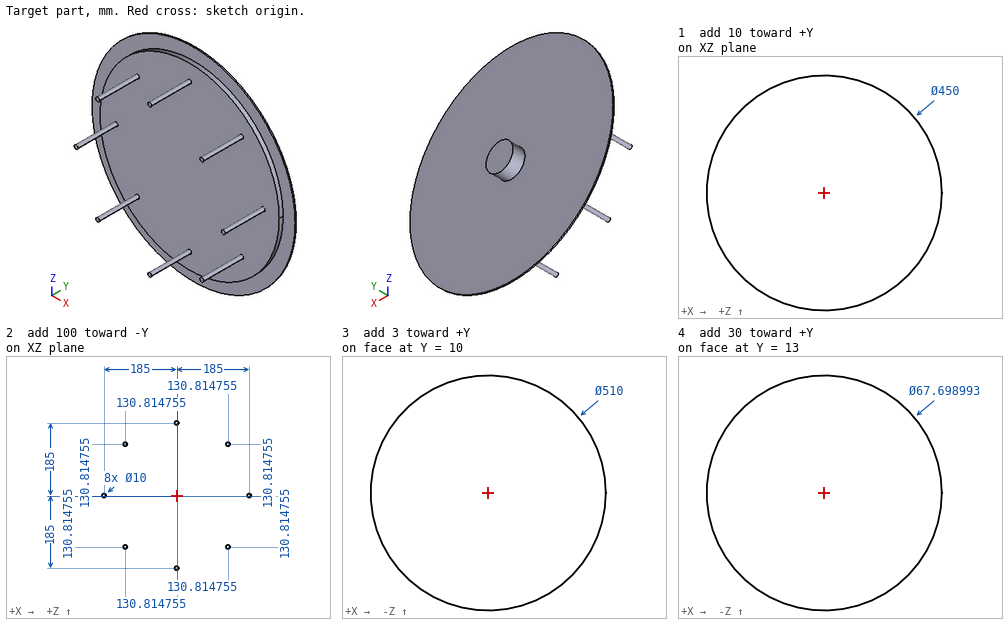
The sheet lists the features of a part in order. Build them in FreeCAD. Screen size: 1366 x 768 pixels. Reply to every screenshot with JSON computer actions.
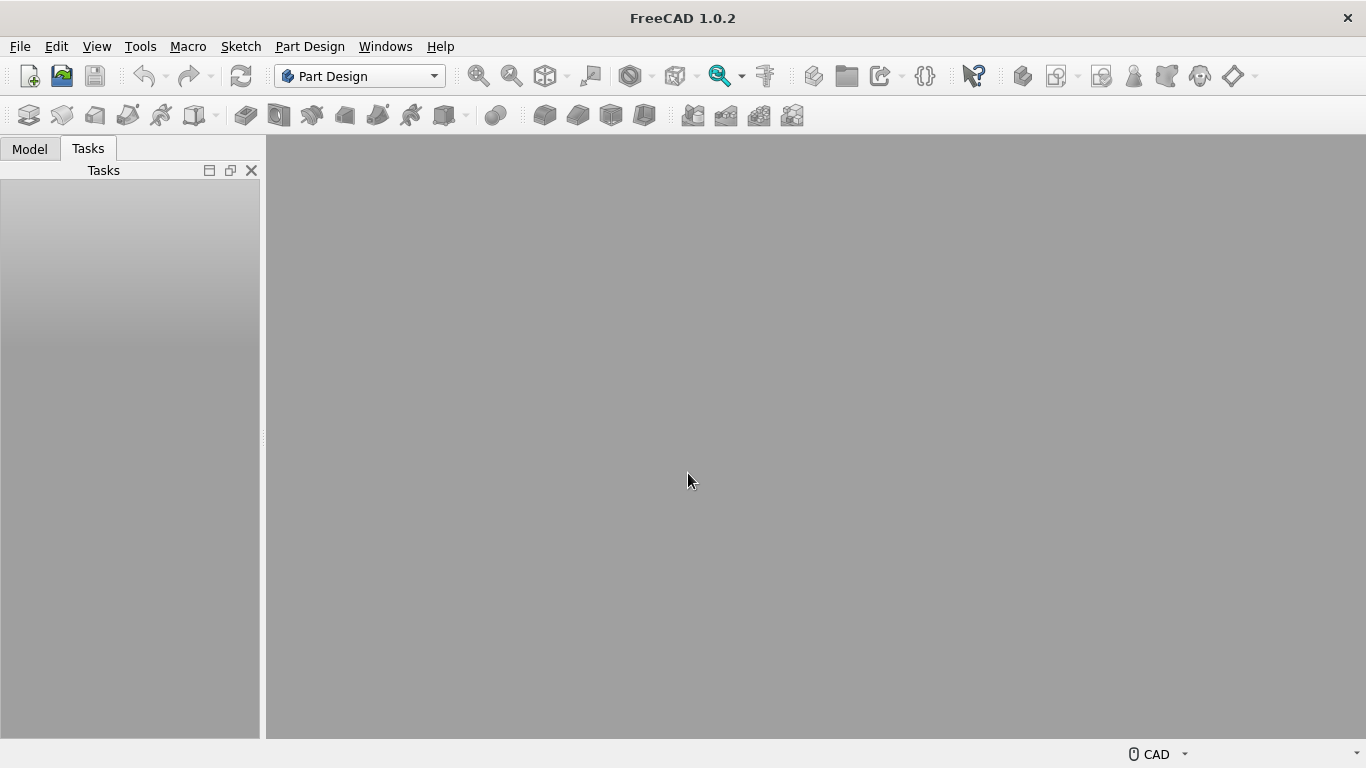
{"action": "left_click", "coordinate": [29, 76]}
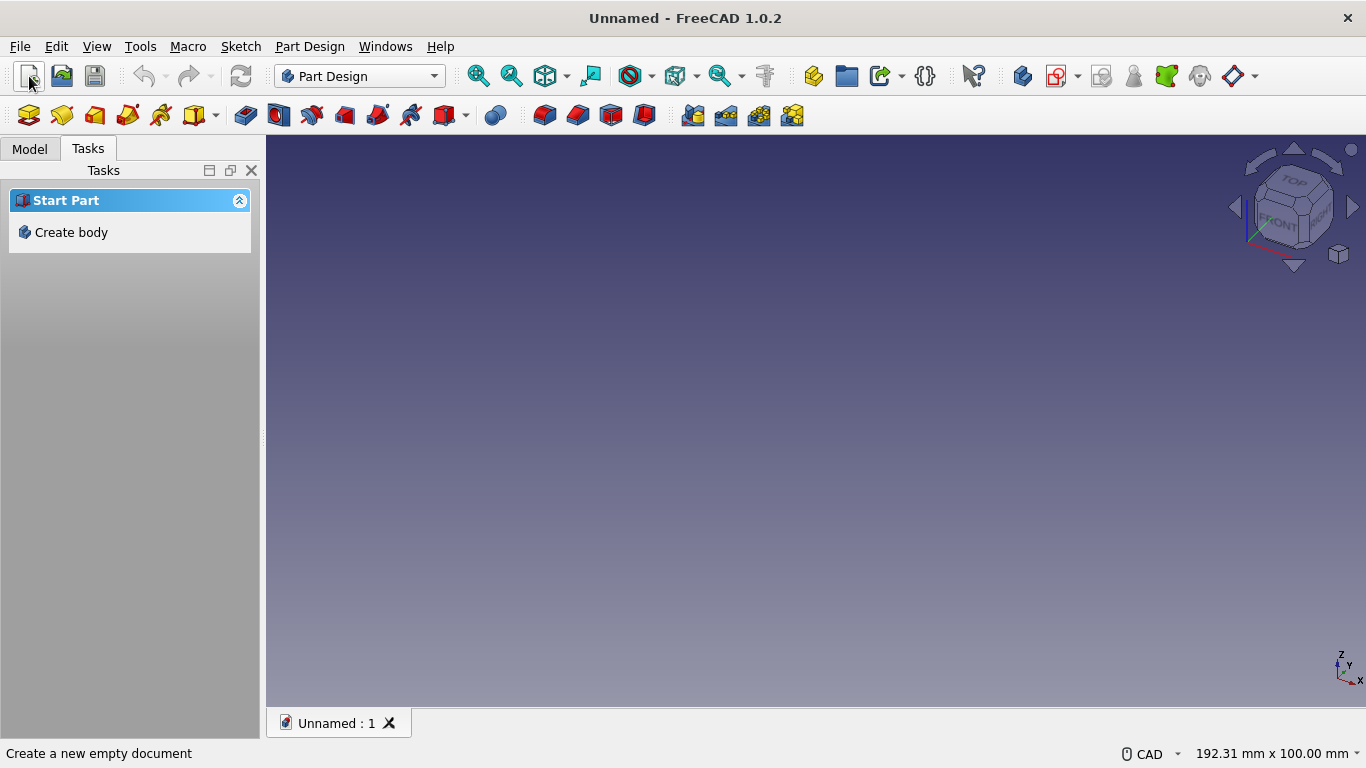
{"action": "left_click", "coordinate": [1056, 76]}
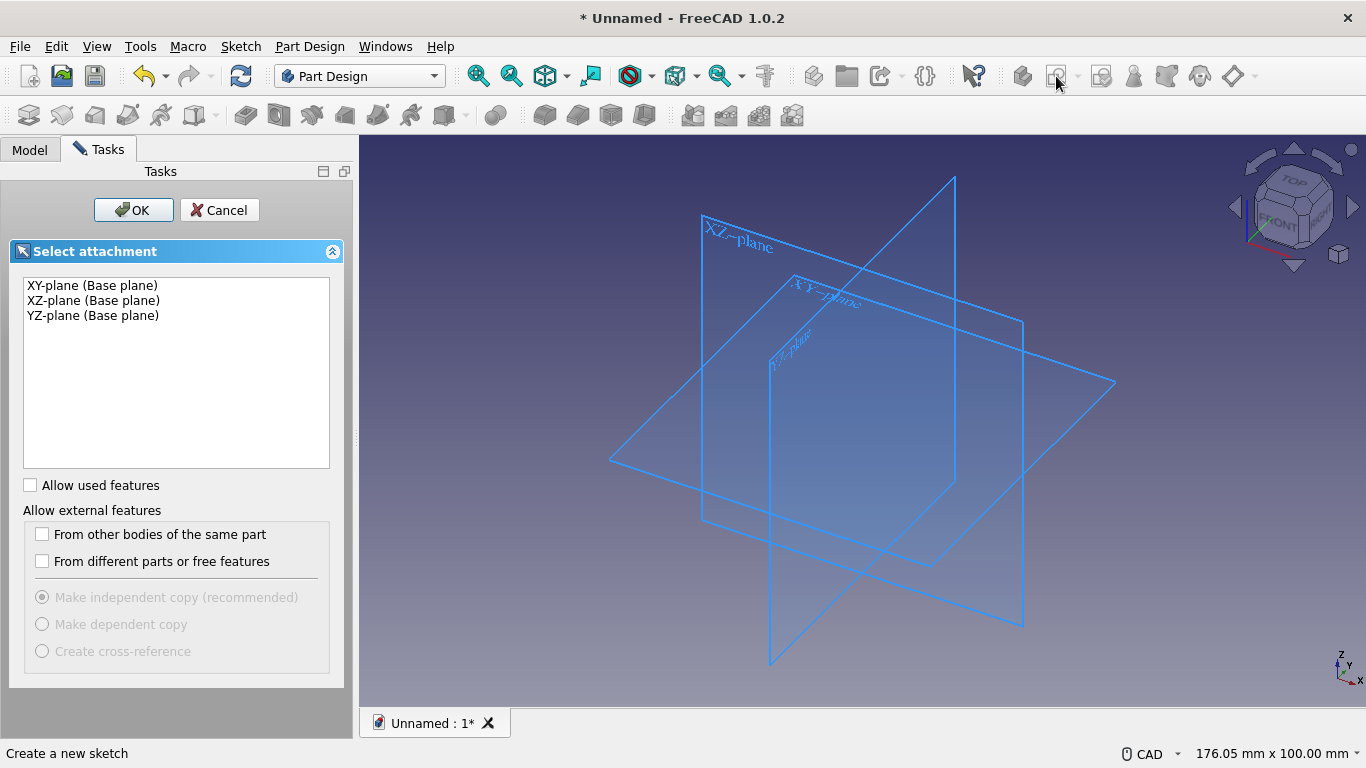
{"action": "left_click", "coordinate": [84, 300]}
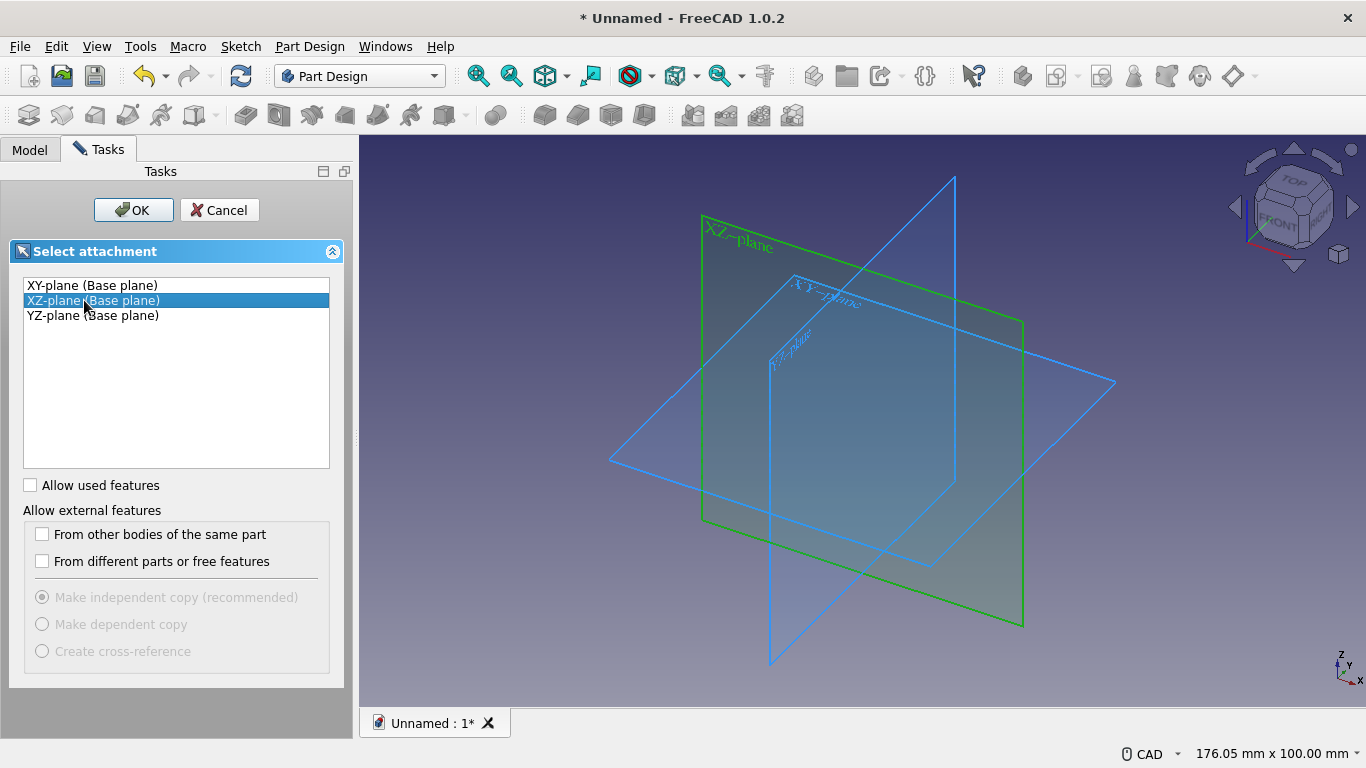
{"action": "left_click", "coordinate": [134, 210]}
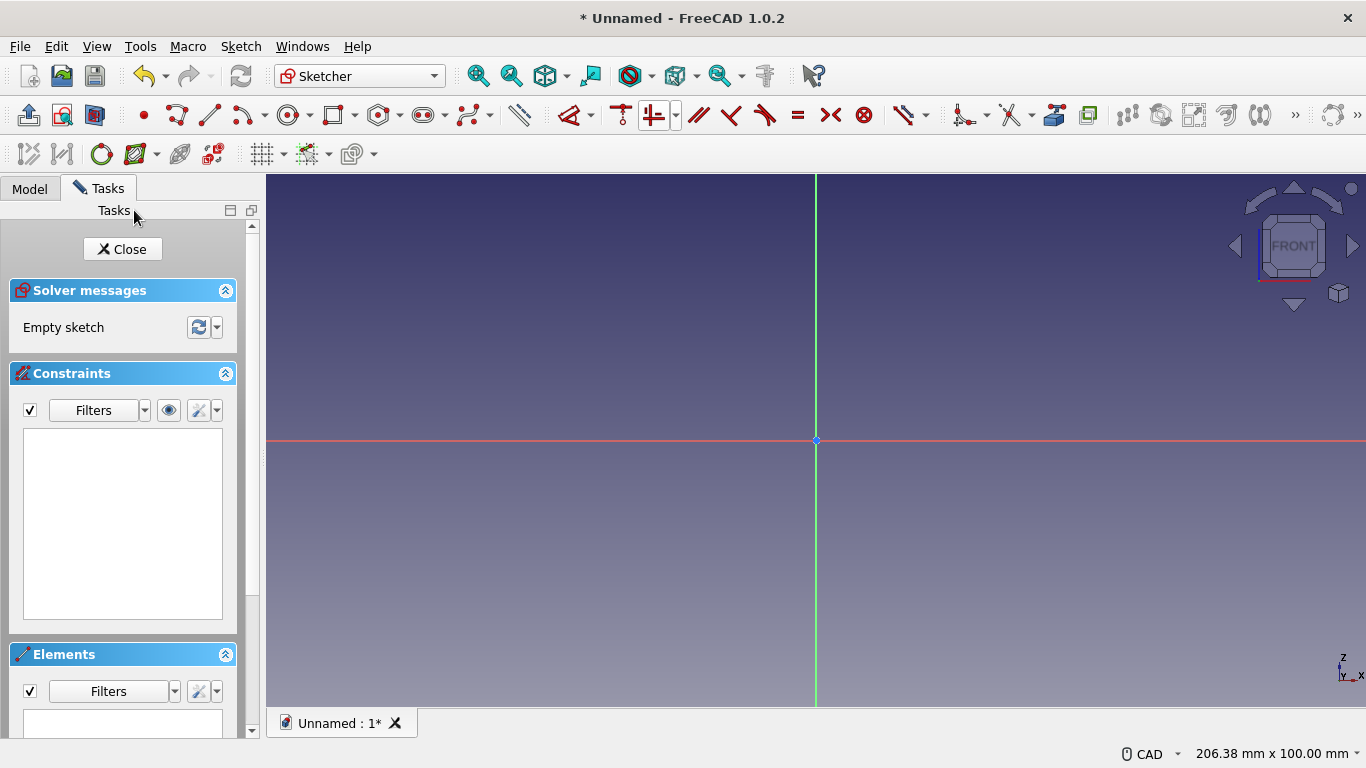
{"action": "scroll", "coordinate": [737, 440], "scroll_direction": "down", "scroll_amount": 10}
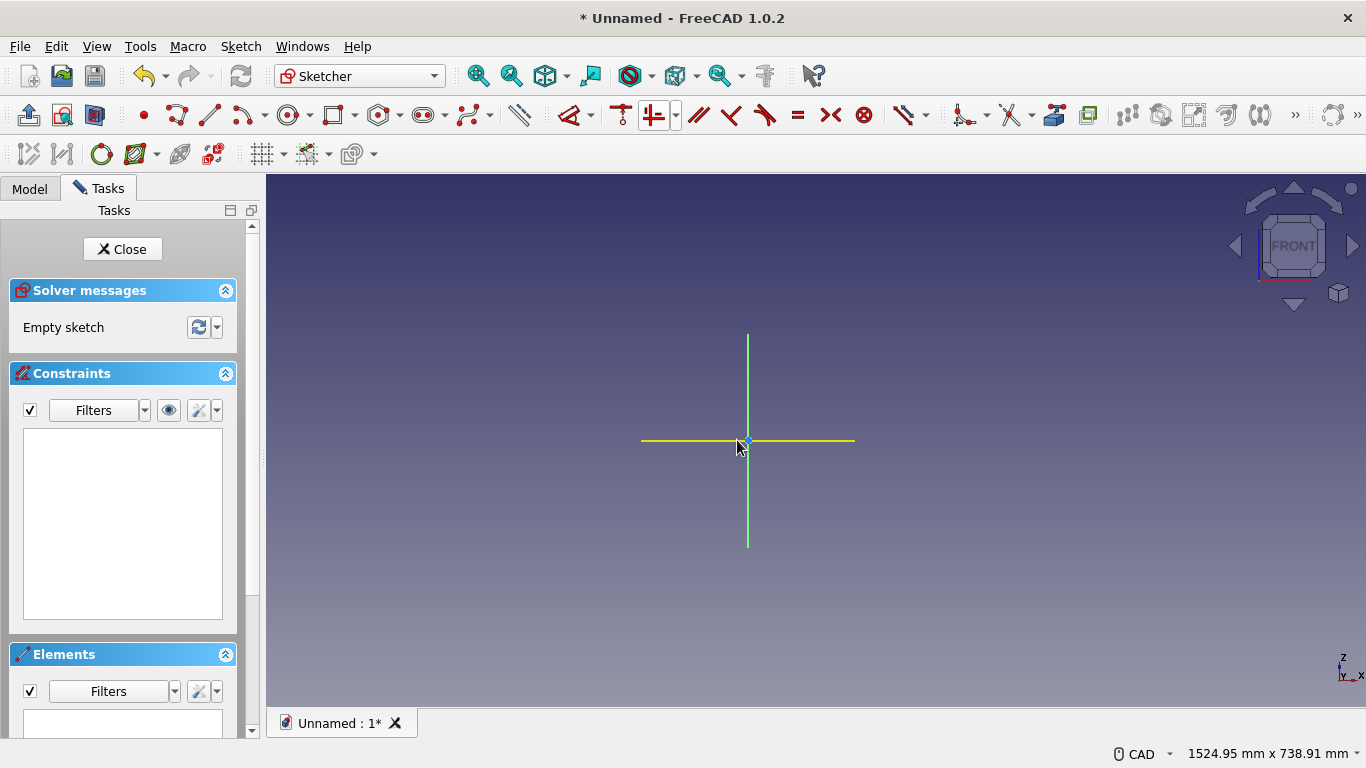
{"action": "left_click", "coordinate": [288, 116]}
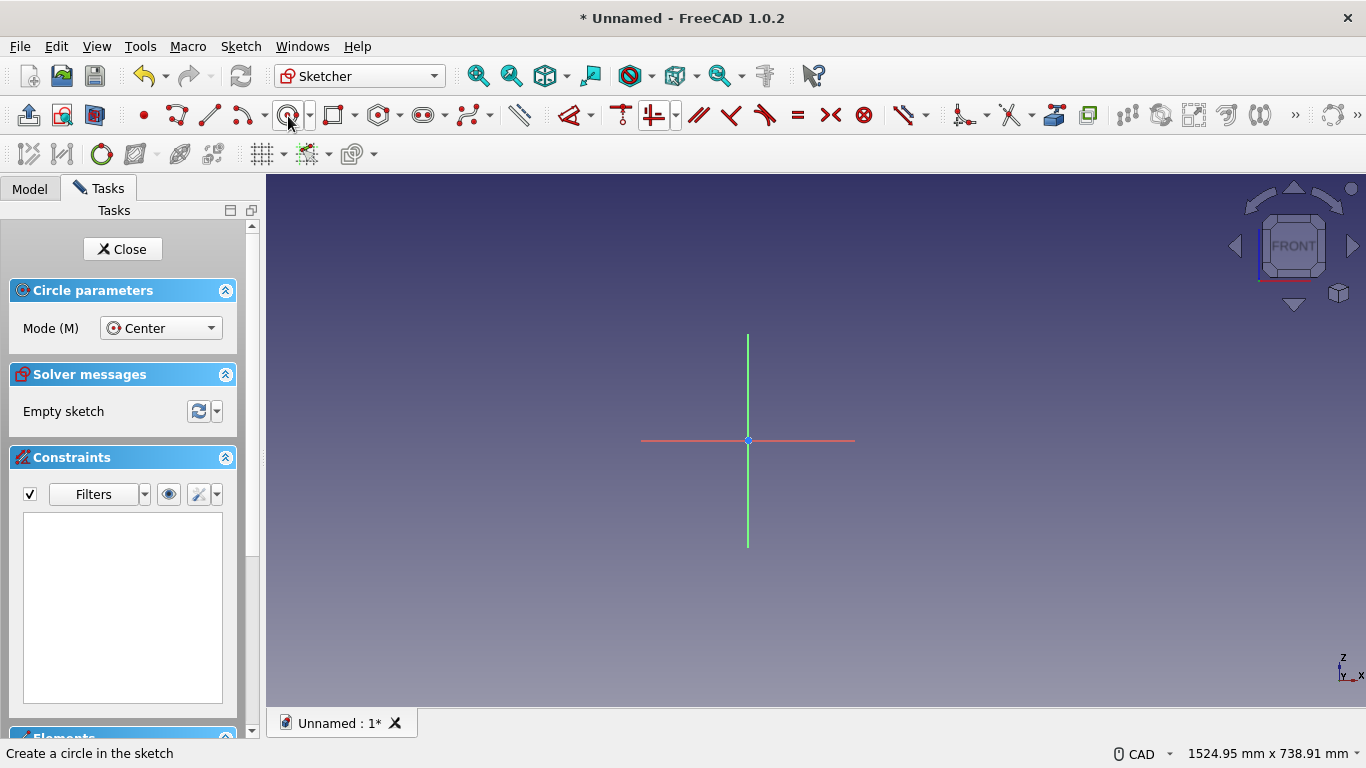
{"action": "left_click", "coordinate": [748, 440]}
{"action": "left_click", "coordinate": [863, 326]}
{"action": "key", "text": "Escape"}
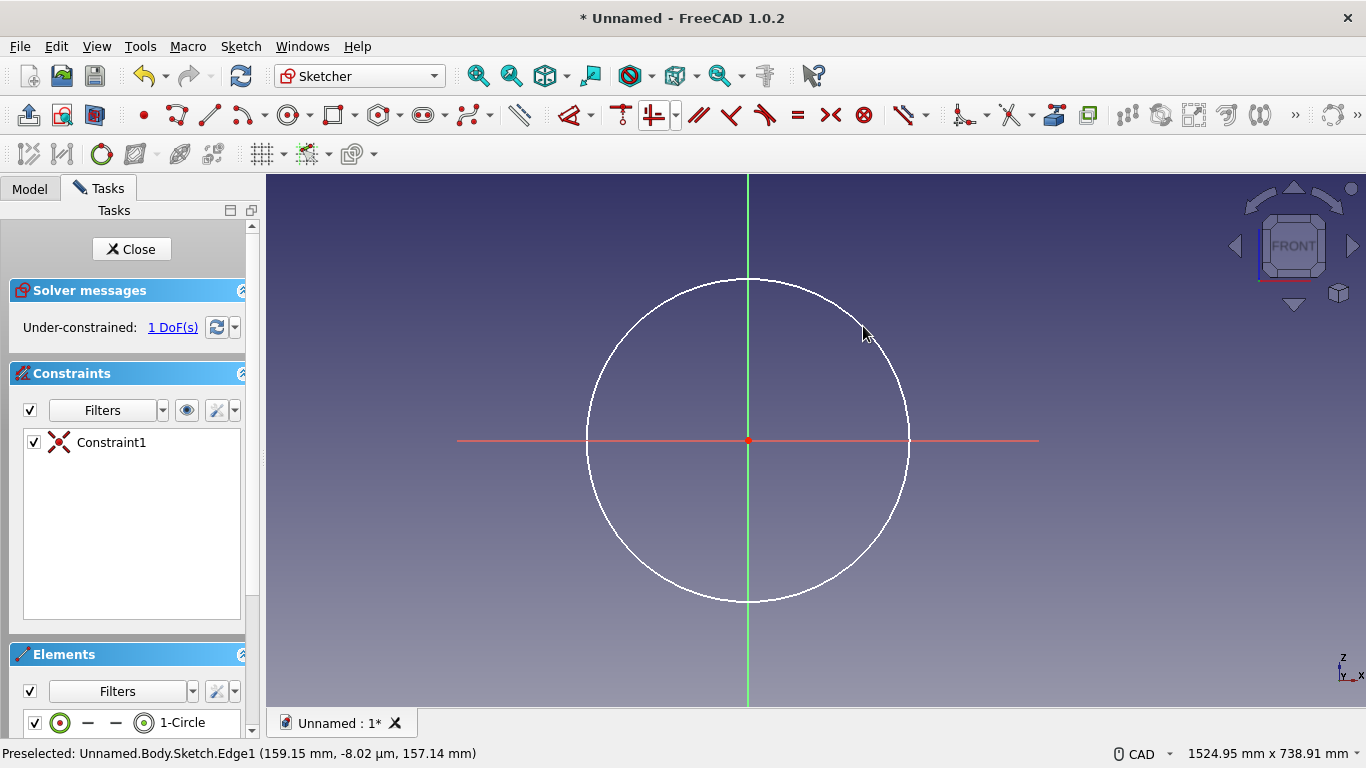
{"action": "left_click", "coordinate": [862, 326]}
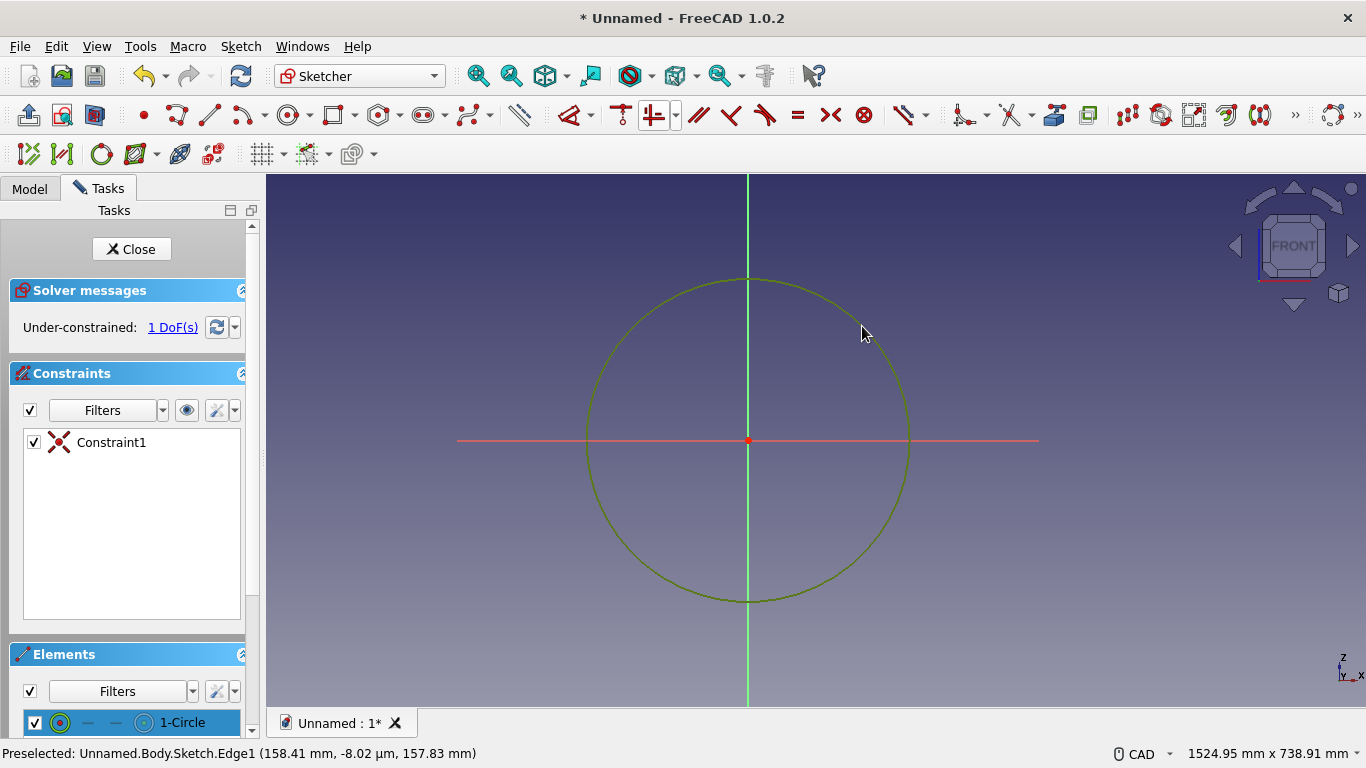
{"action": "left_click", "coordinate": [590, 116]}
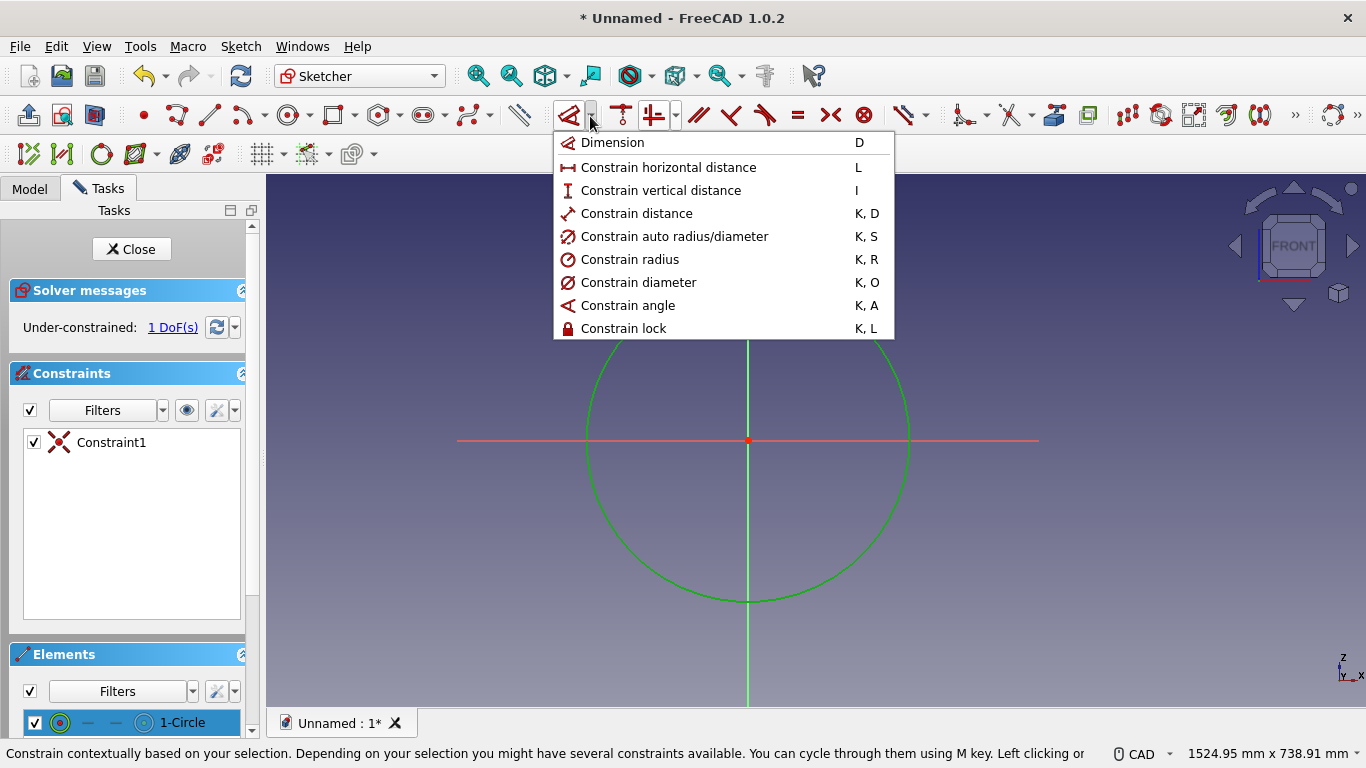
{"action": "left_click", "coordinate": [724, 282]}